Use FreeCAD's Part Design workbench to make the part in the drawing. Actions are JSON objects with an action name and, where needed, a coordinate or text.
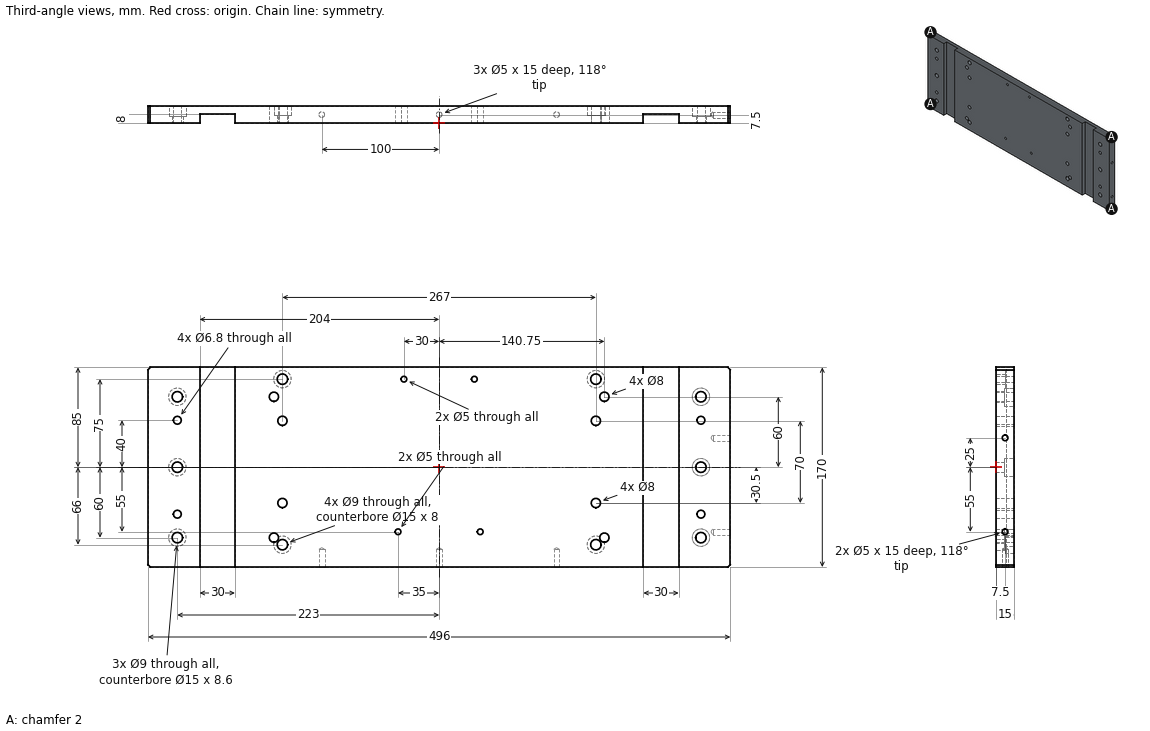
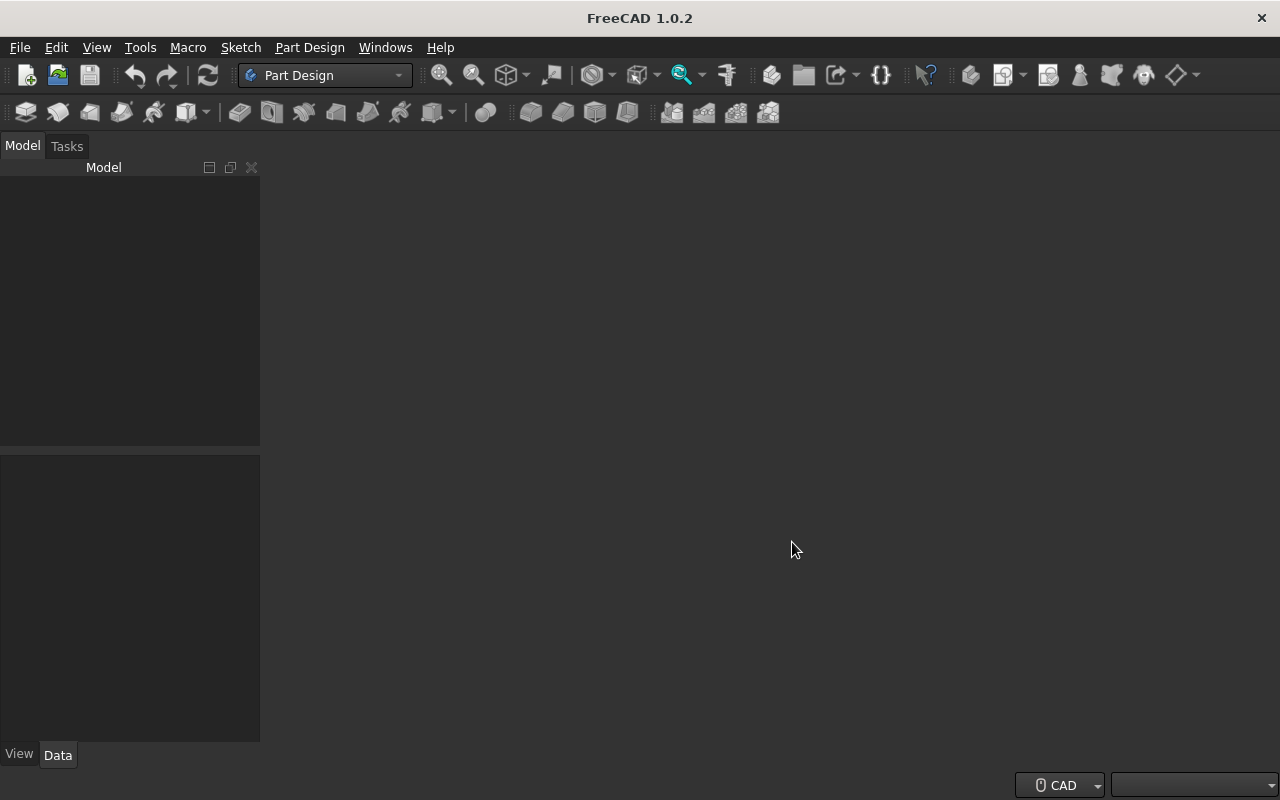
{"action": "left_click", "coordinate": [26, 76]}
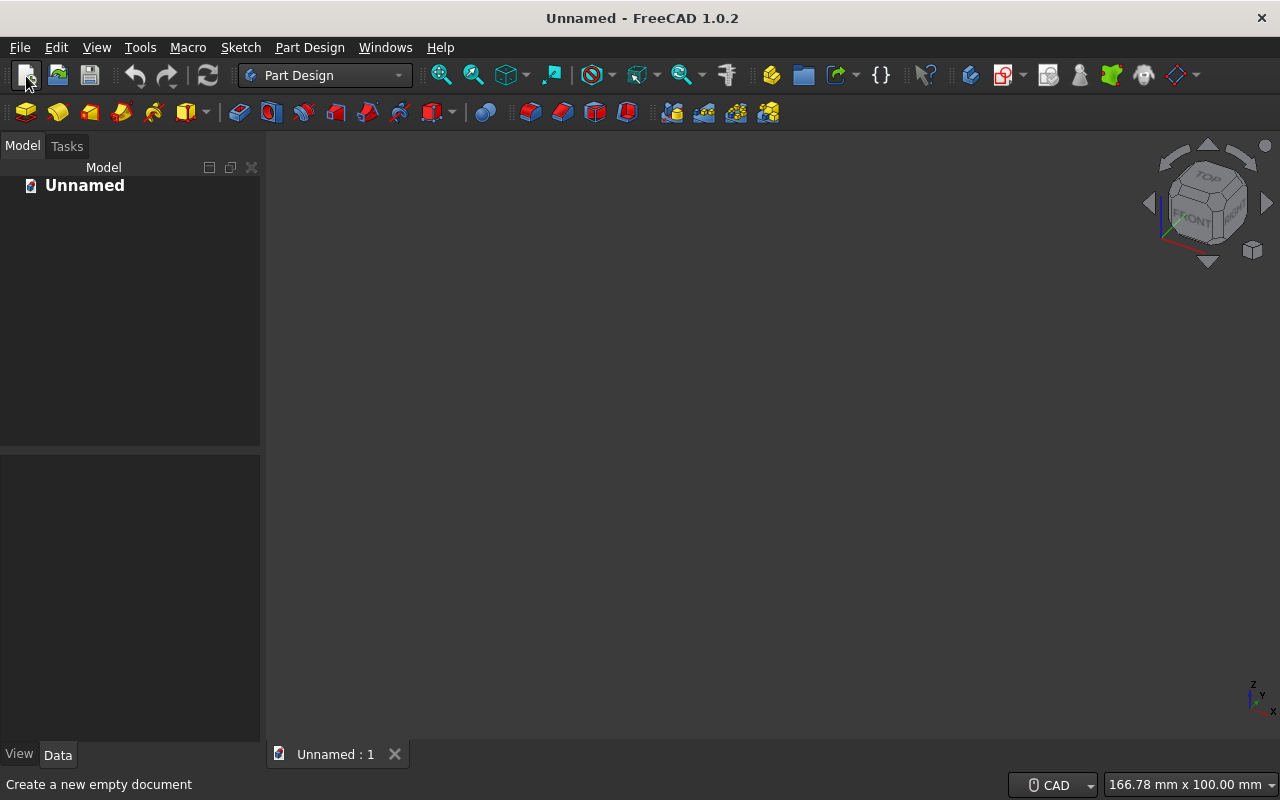
{"action": "left_click", "coordinate": [1004, 76]}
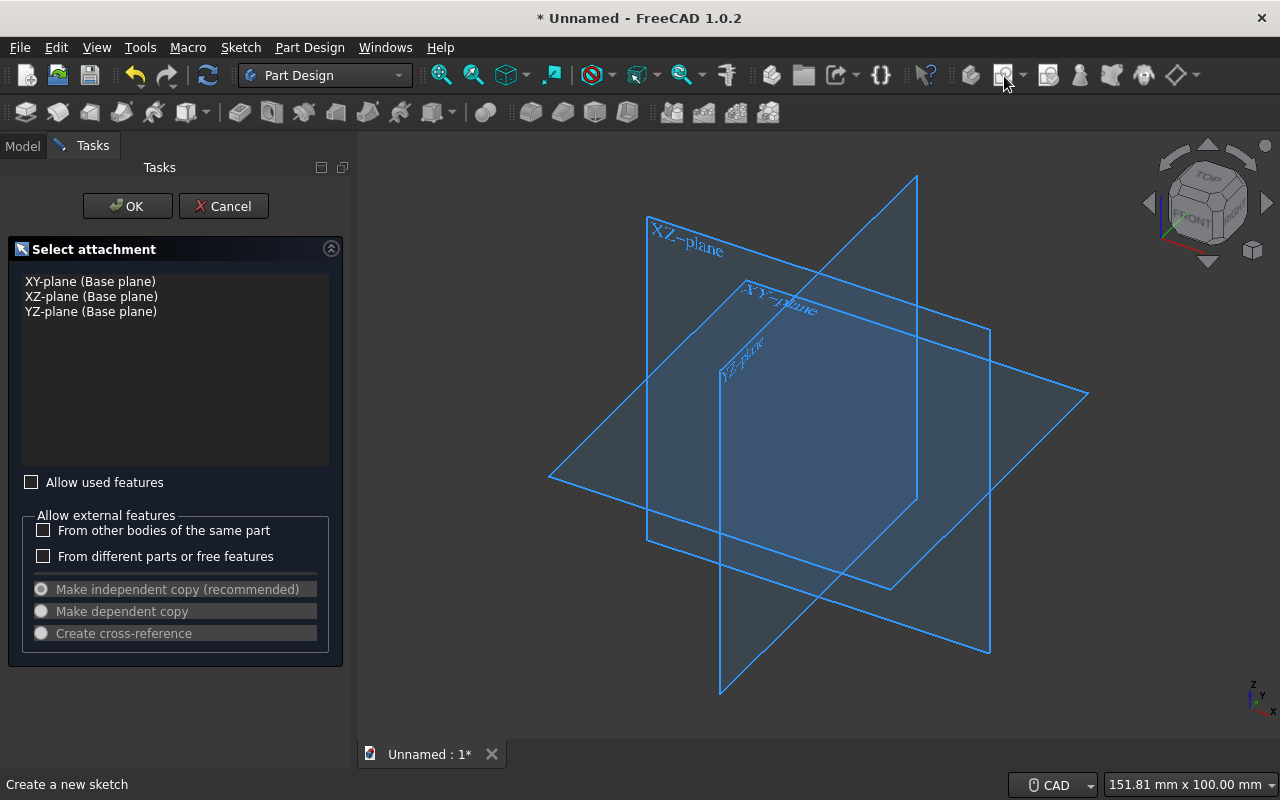
{"action": "left_click", "coordinate": [82, 296]}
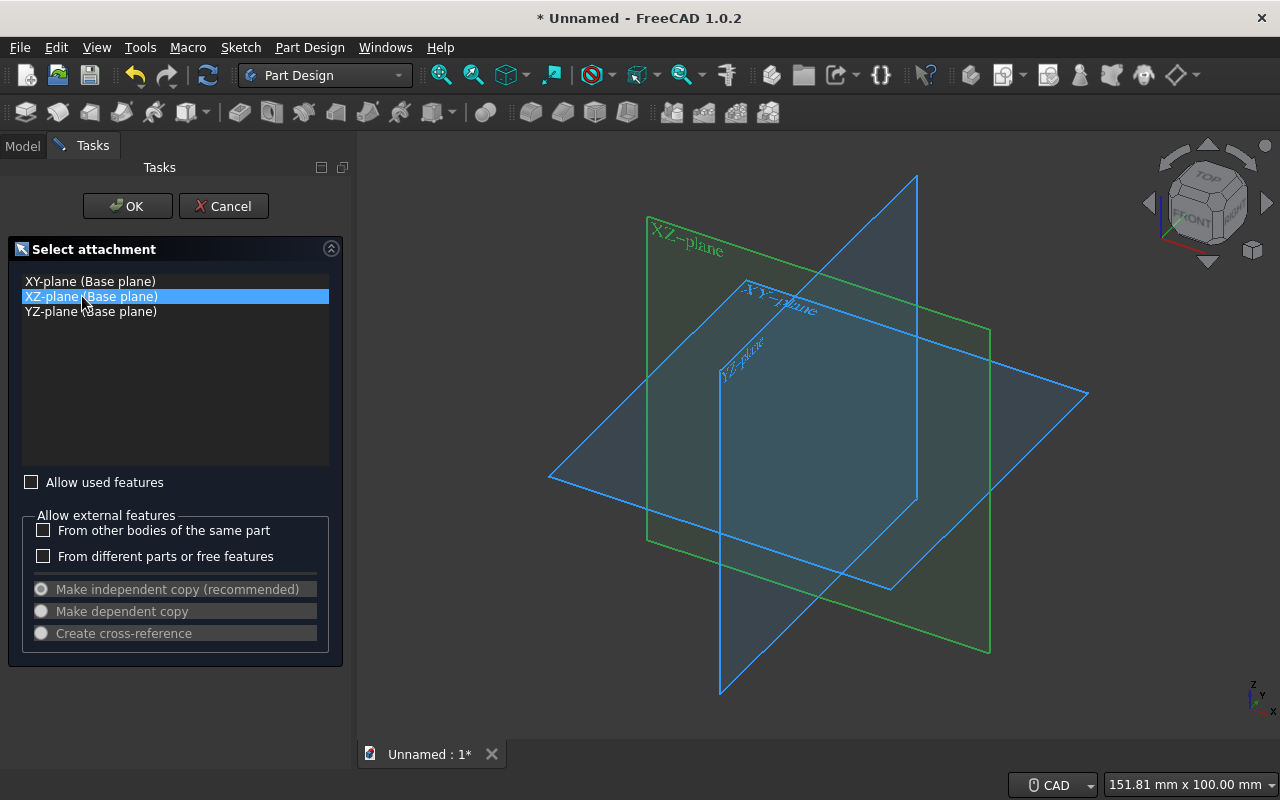
{"action": "left_click", "coordinate": [128, 206]}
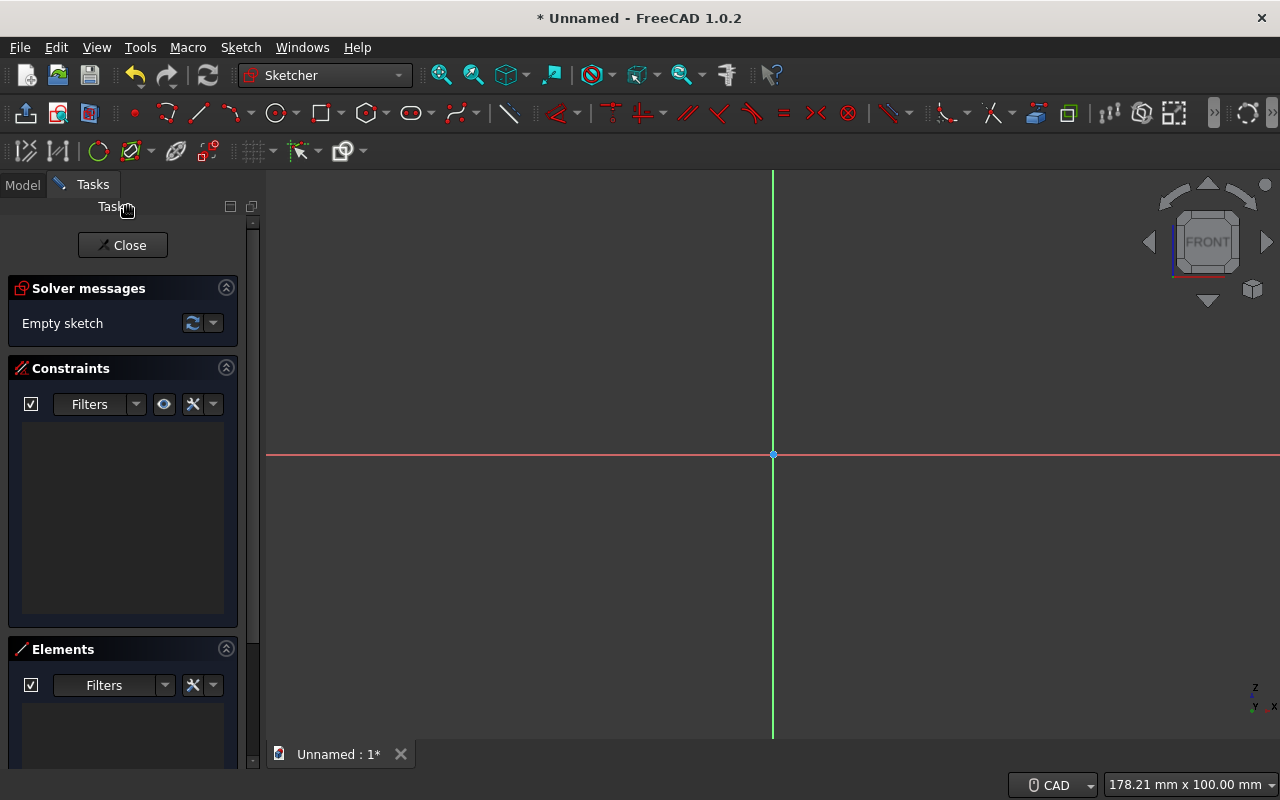
{"action": "scroll", "coordinate": [687, 454], "scroll_direction": "down", "scroll_amount": 8}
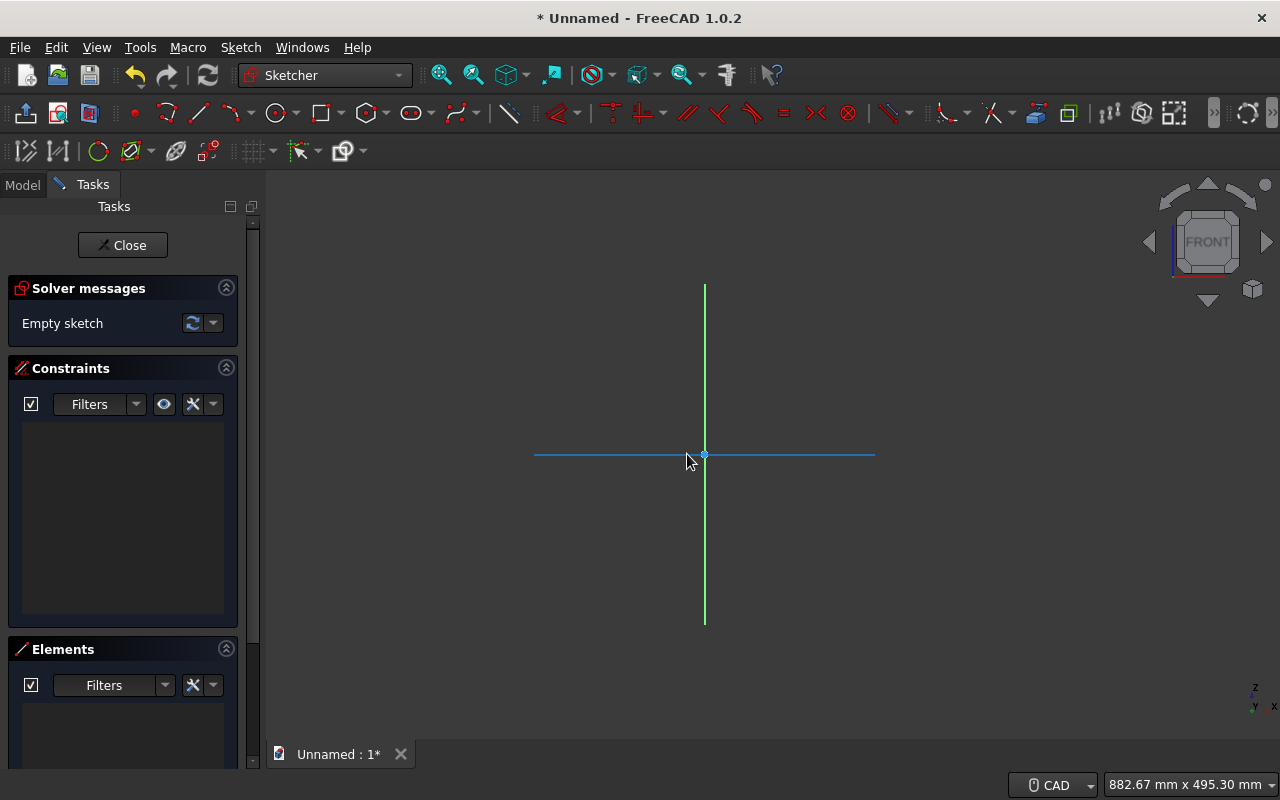
{"action": "left_click", "coordinate": [344, 114]}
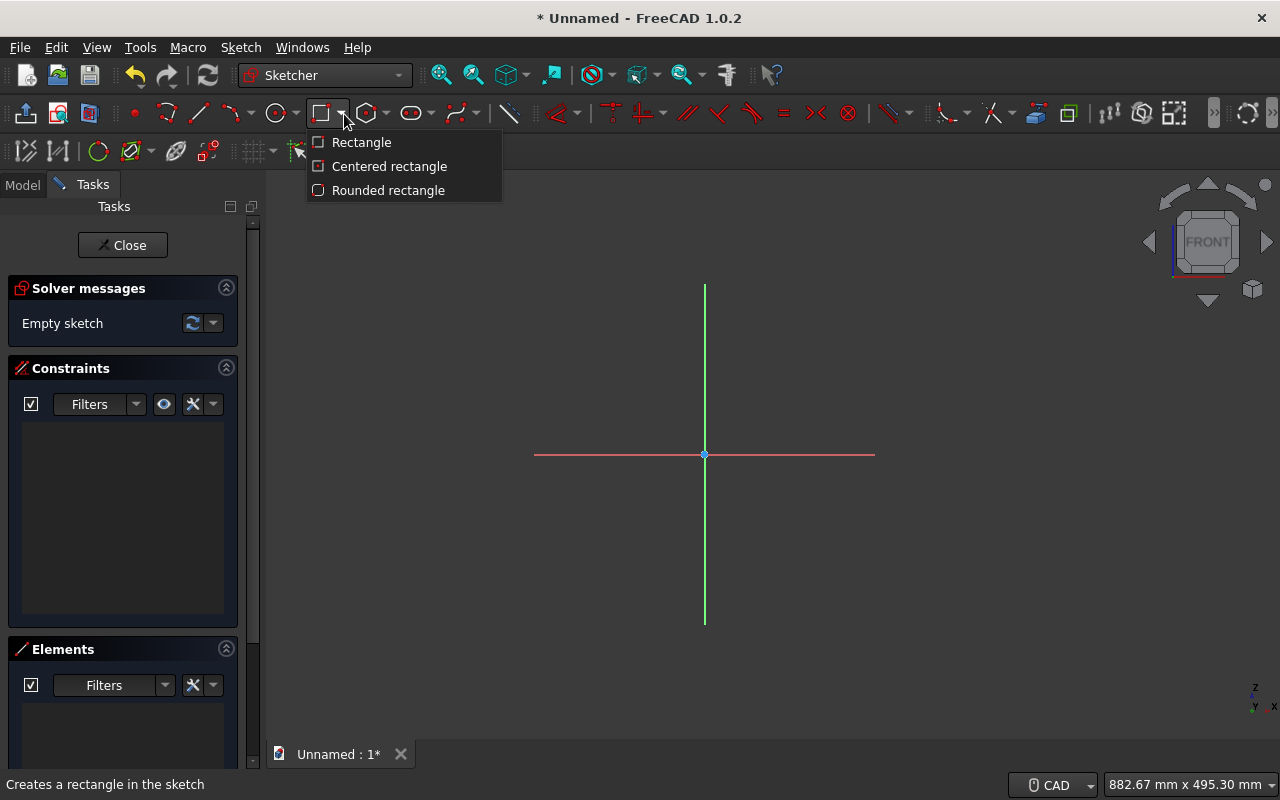
{"action": "left_click", "coordinate": [404, 166]}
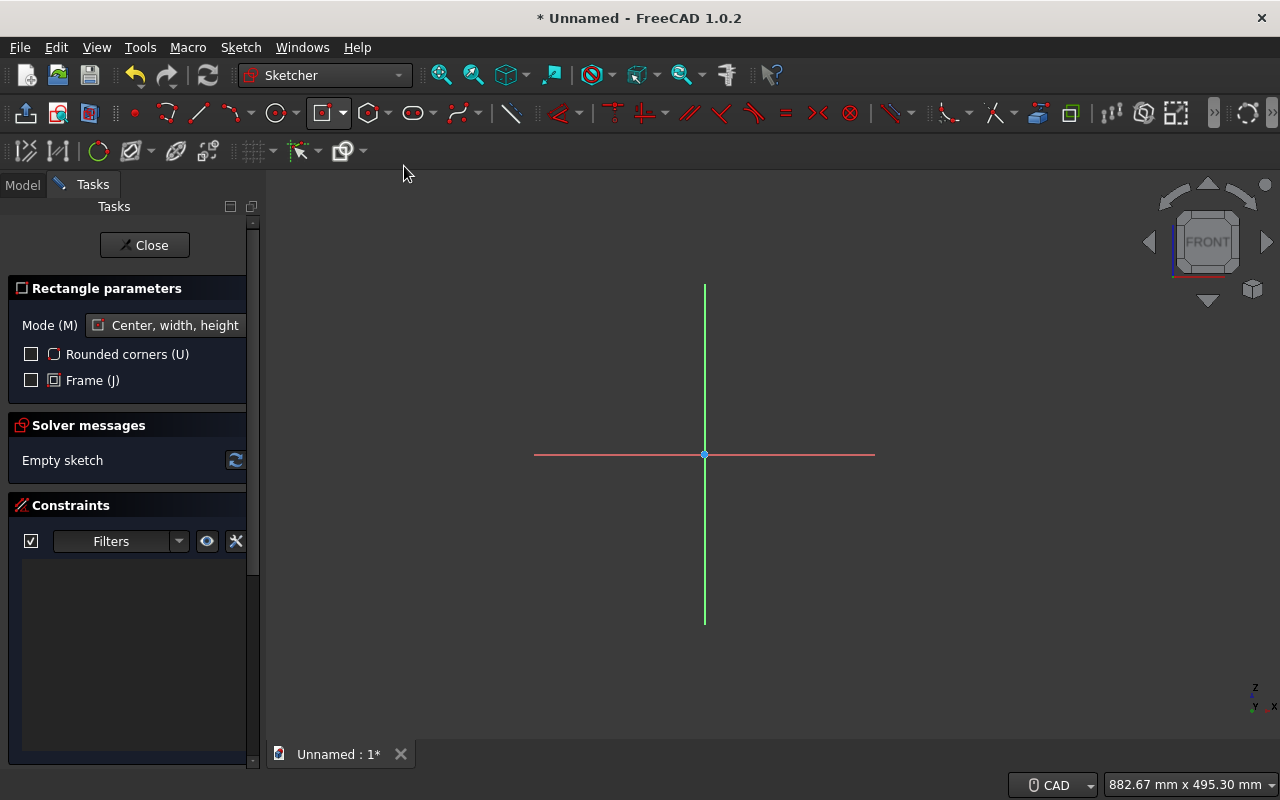
{"action": "left_click", "coordinate": [705, 454]}
{"action": "mouse_move", "coordinate": [990, 357]}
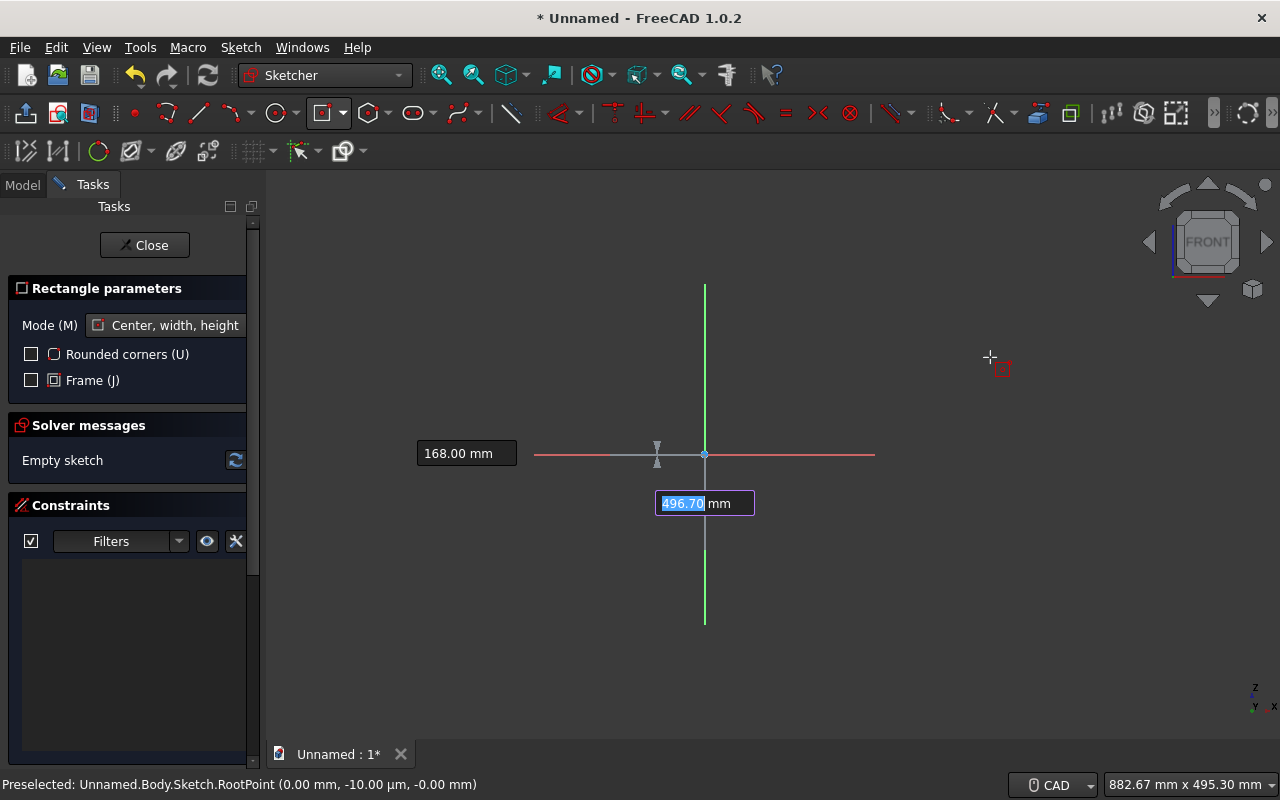
{"action": "type", "text": "496"}
{"action": "key", "text": "Tab"}
{"action": "type", "text": "170"}
{"action": "key", "text": "Return"}
{"action": "key", "text": "Escape"}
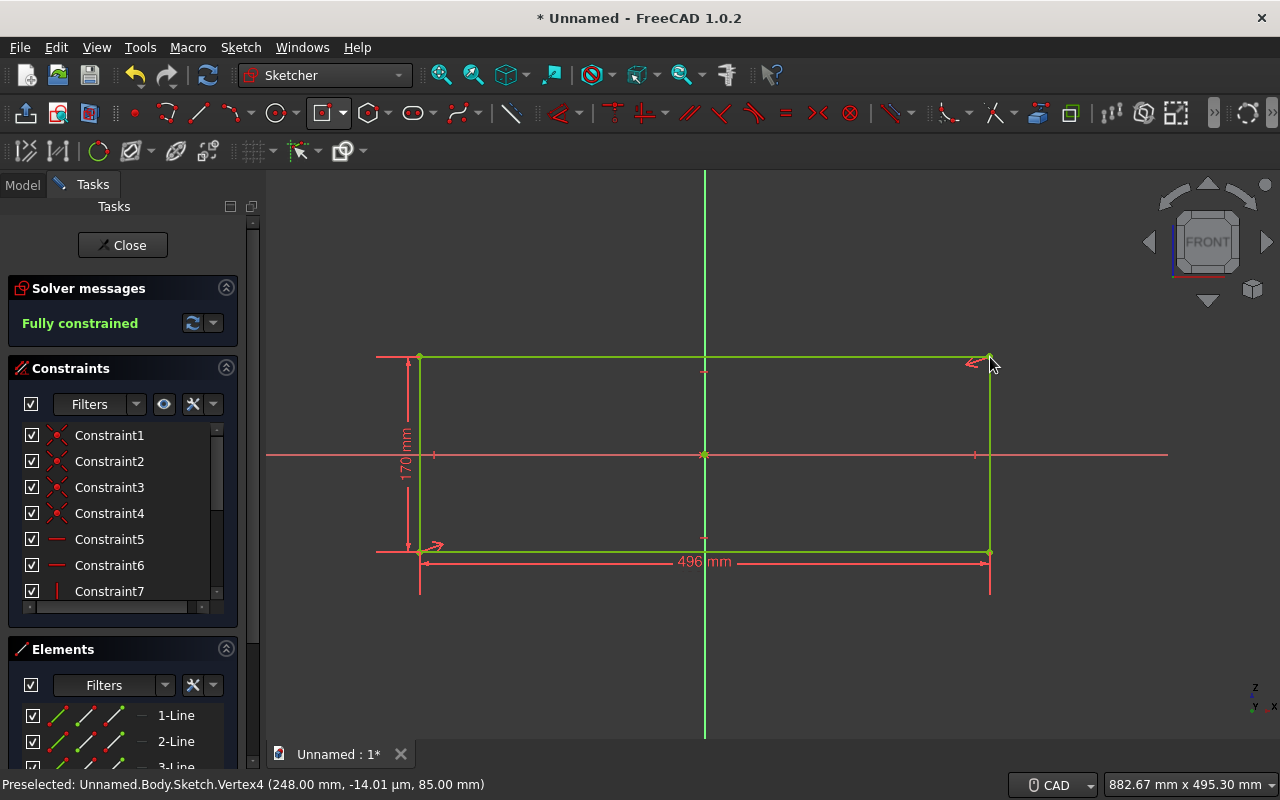
{"action": "left_click", "coordinate": [123, 245]}